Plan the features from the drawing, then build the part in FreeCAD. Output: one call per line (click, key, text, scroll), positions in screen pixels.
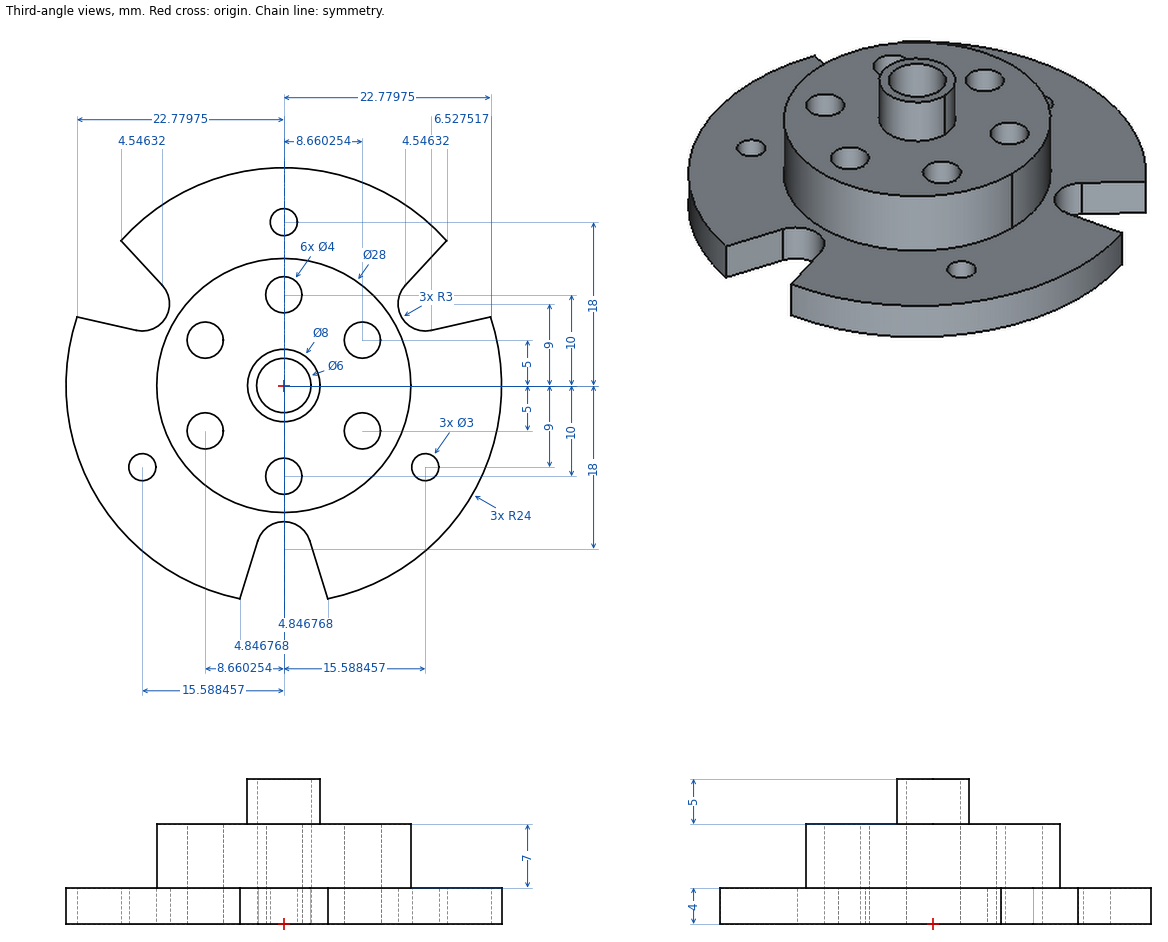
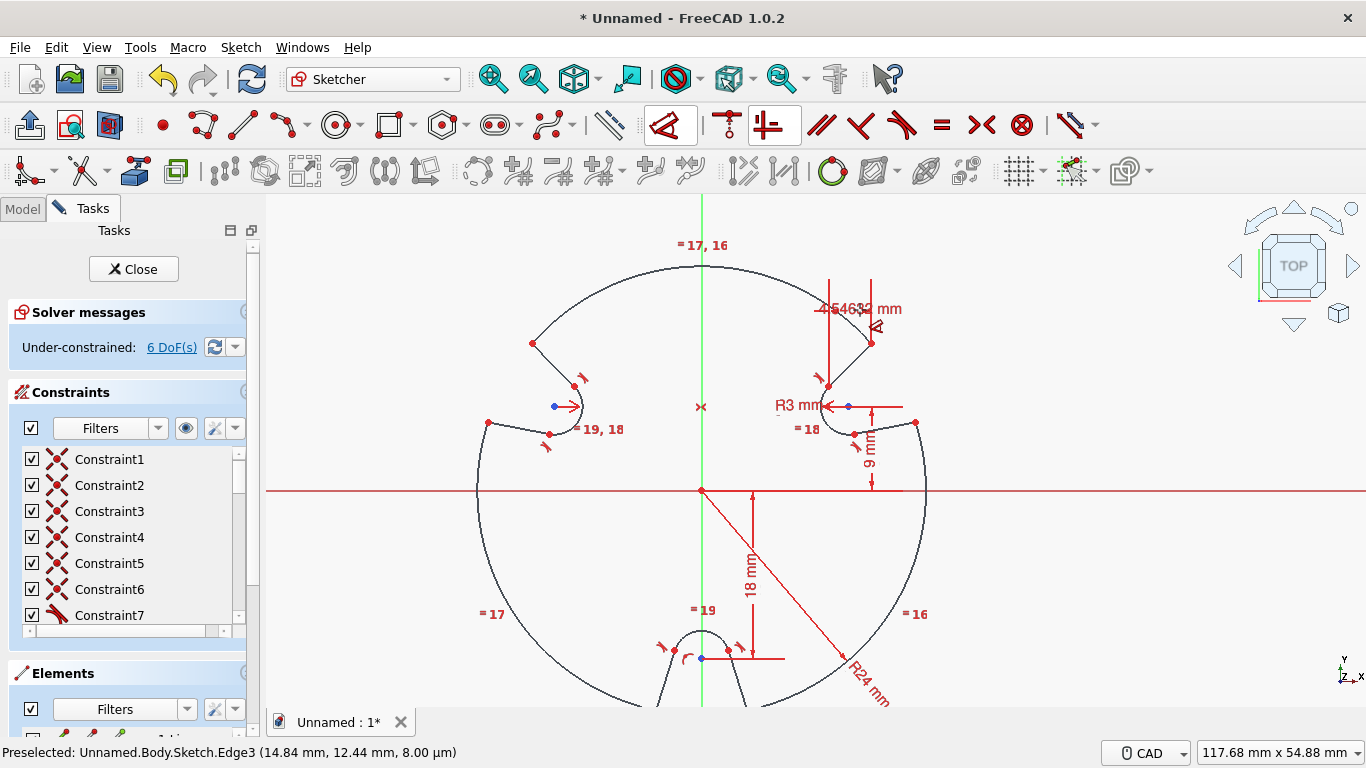
click(545, 357)
click(543, 310)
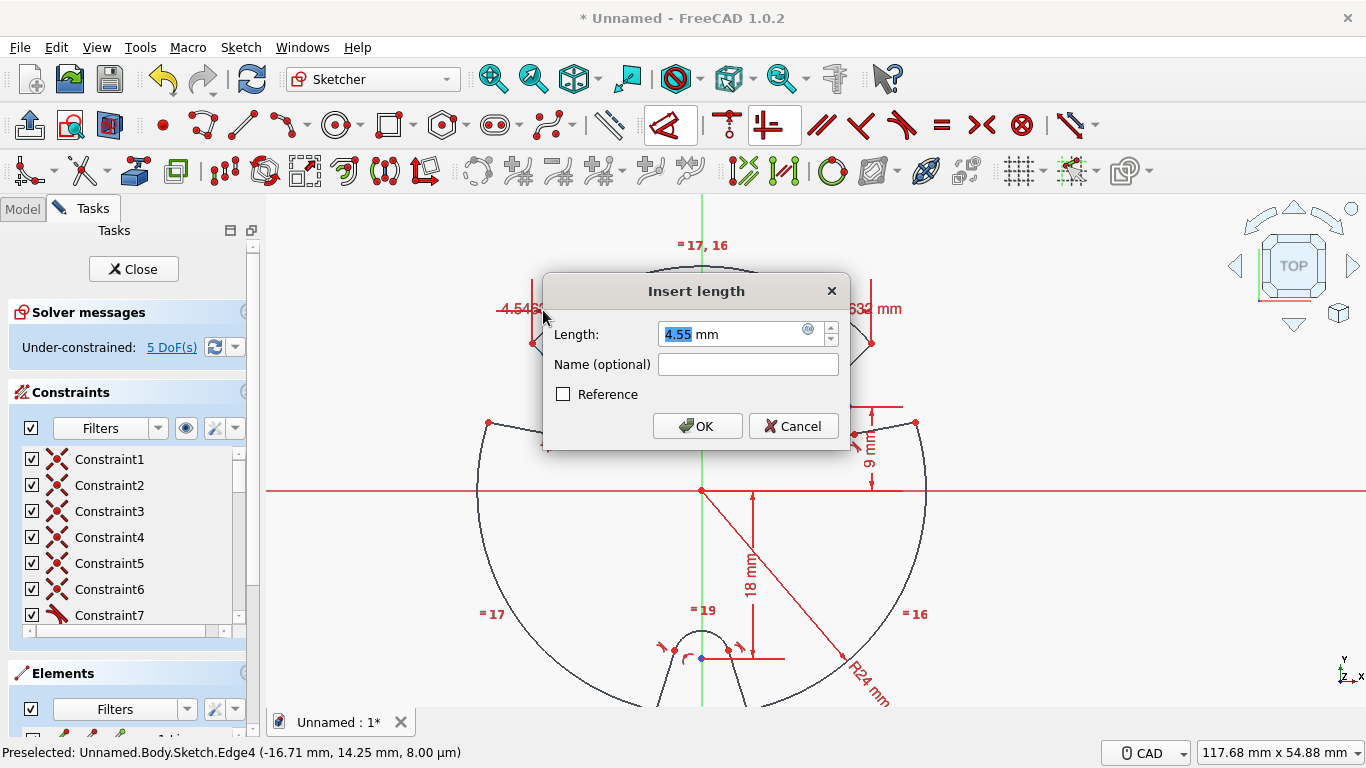
text(4.54632)
key(Return)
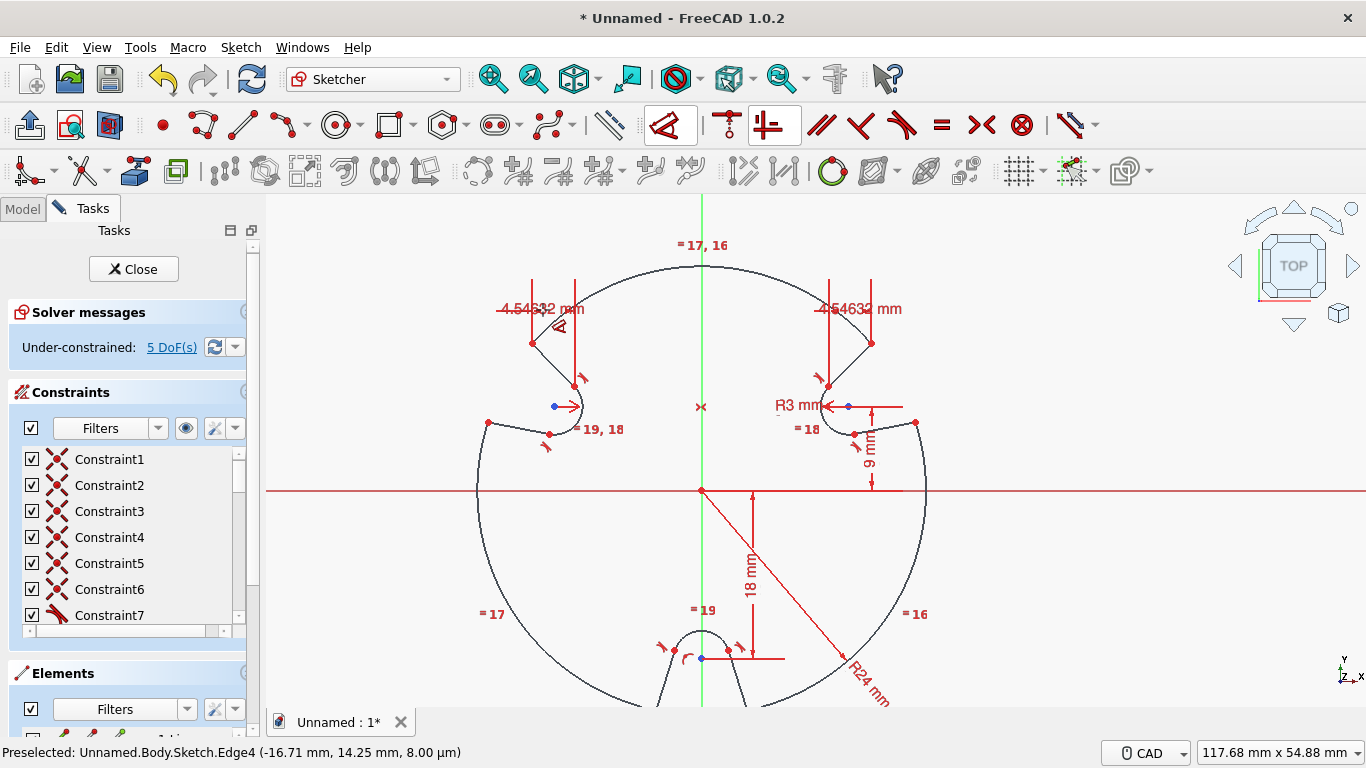
scroll(841, 373, down, 2)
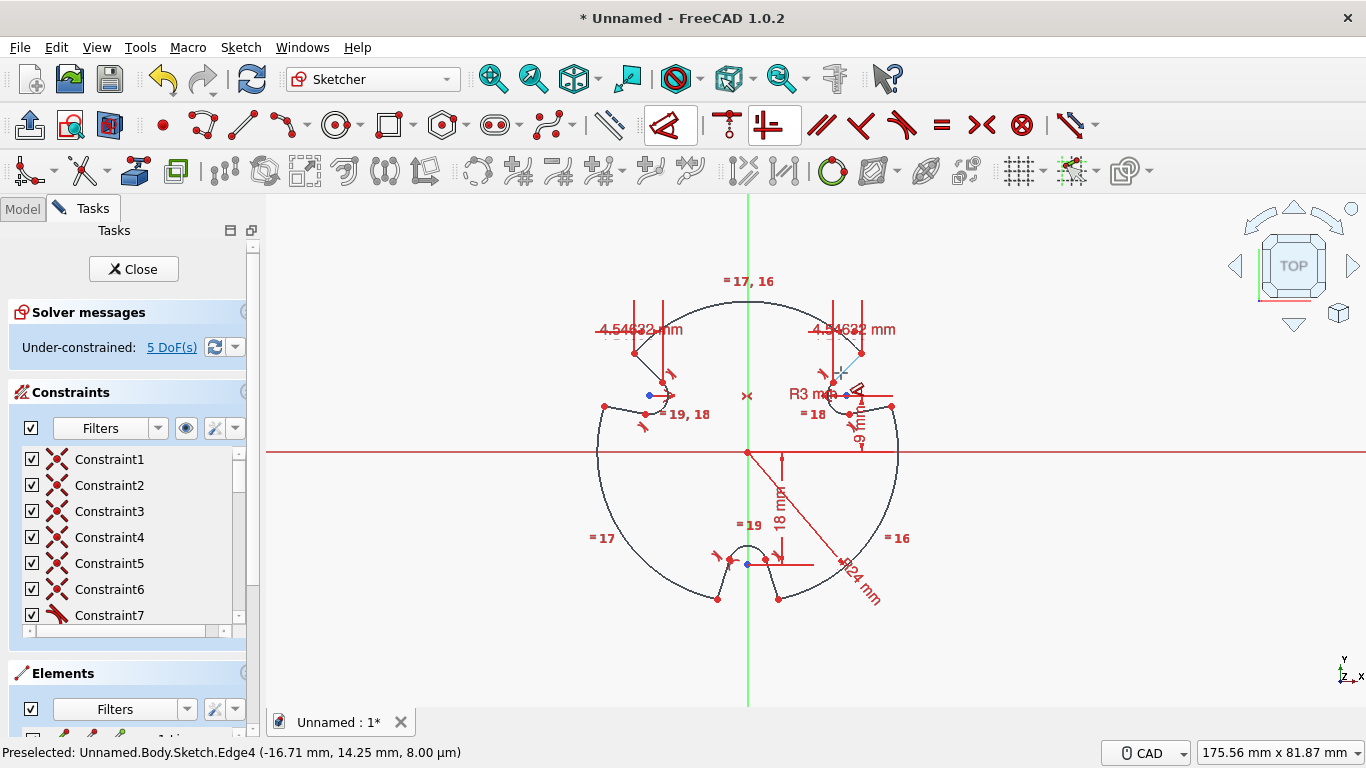
scroll(778, 599, up, 2)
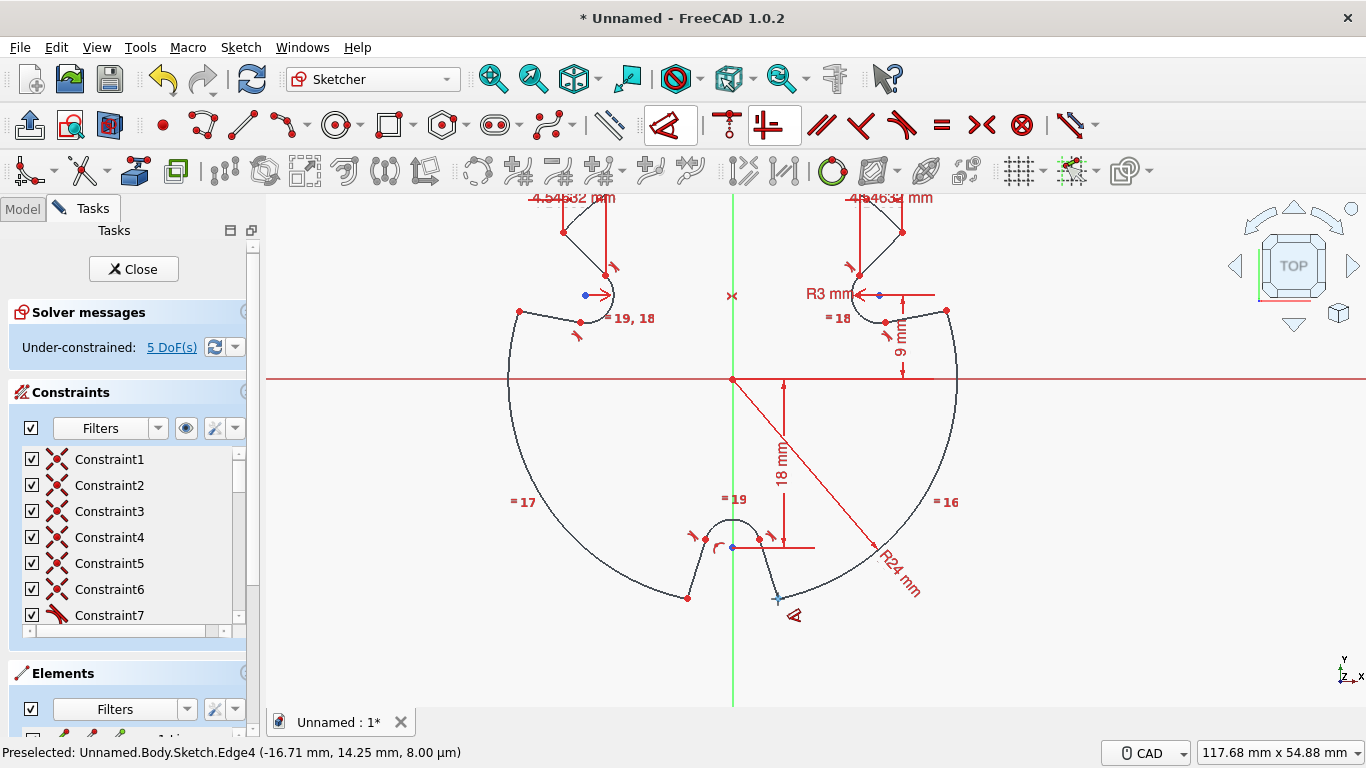
click(778, 599)
click(755, 633)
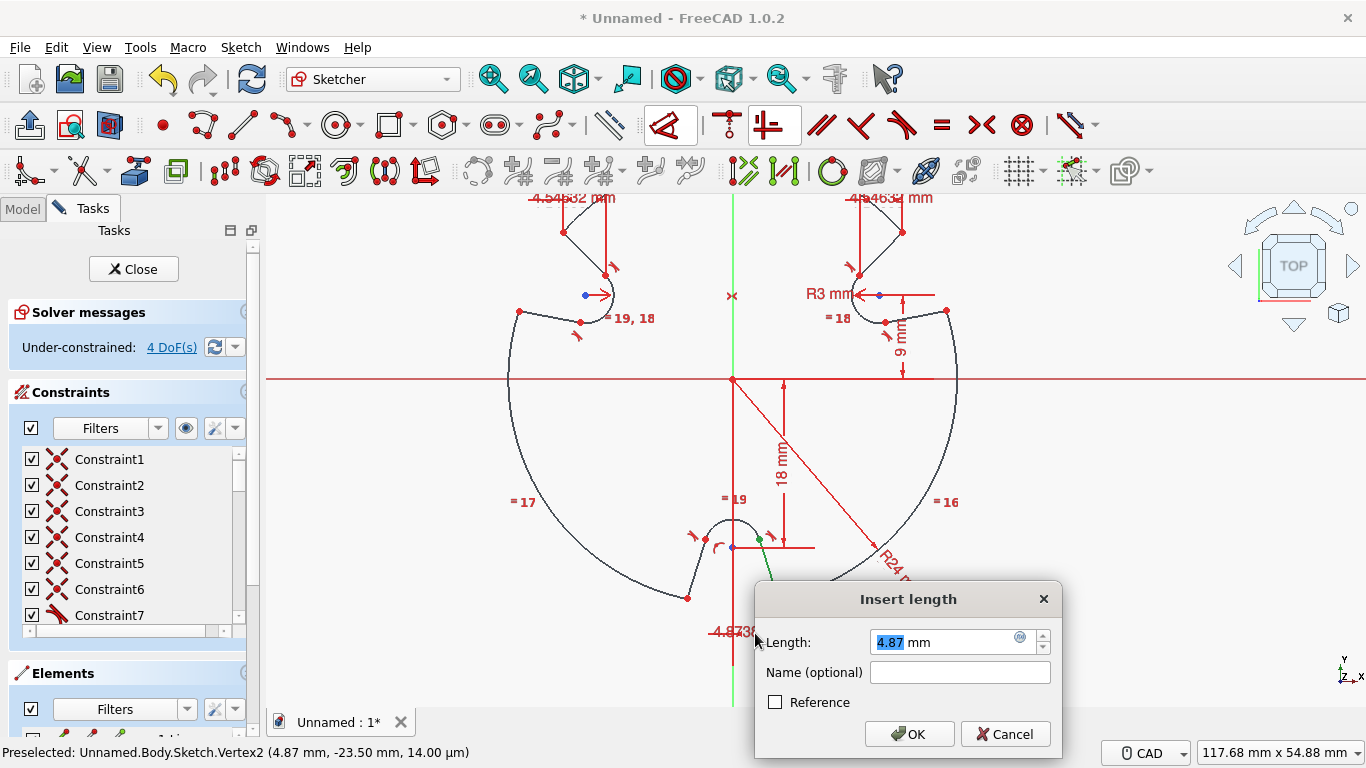
text(4.846768)
key(Return)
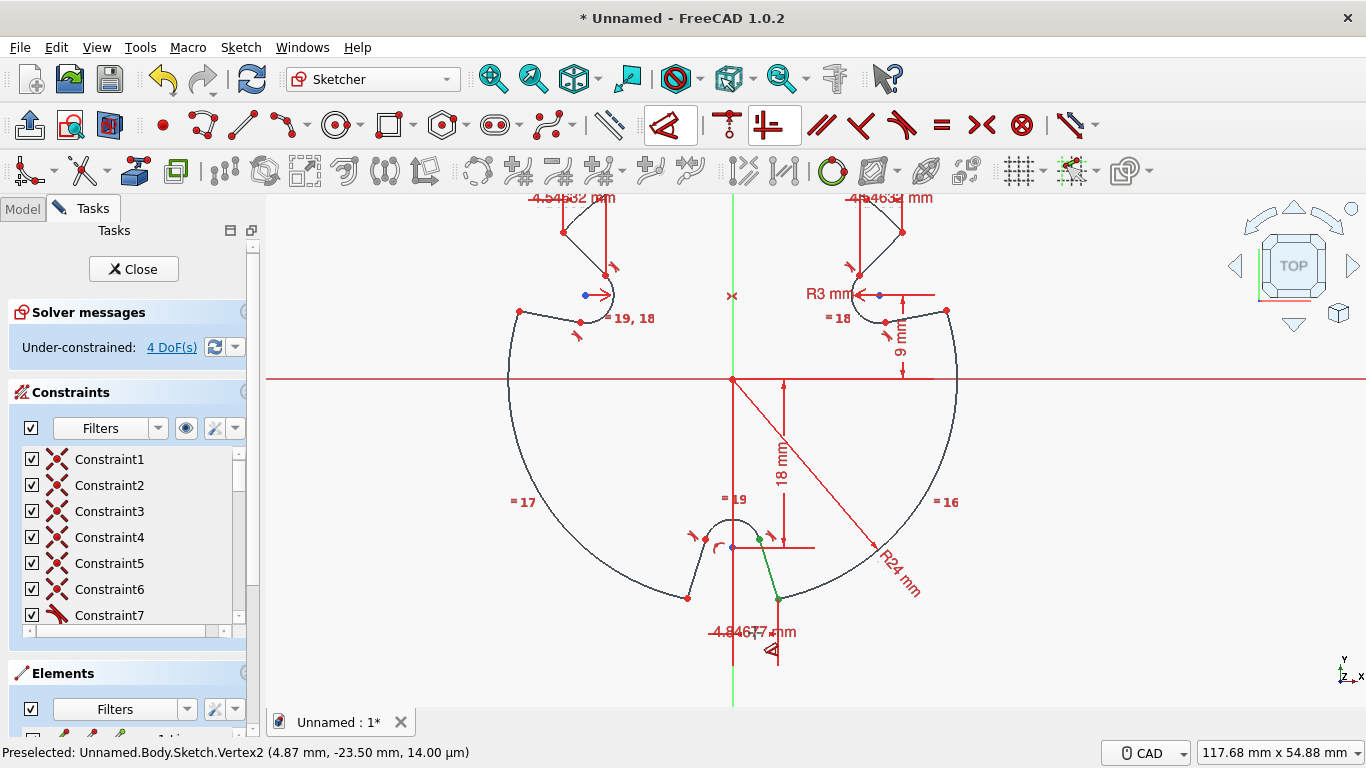
click(946, 311)
click(840, 277)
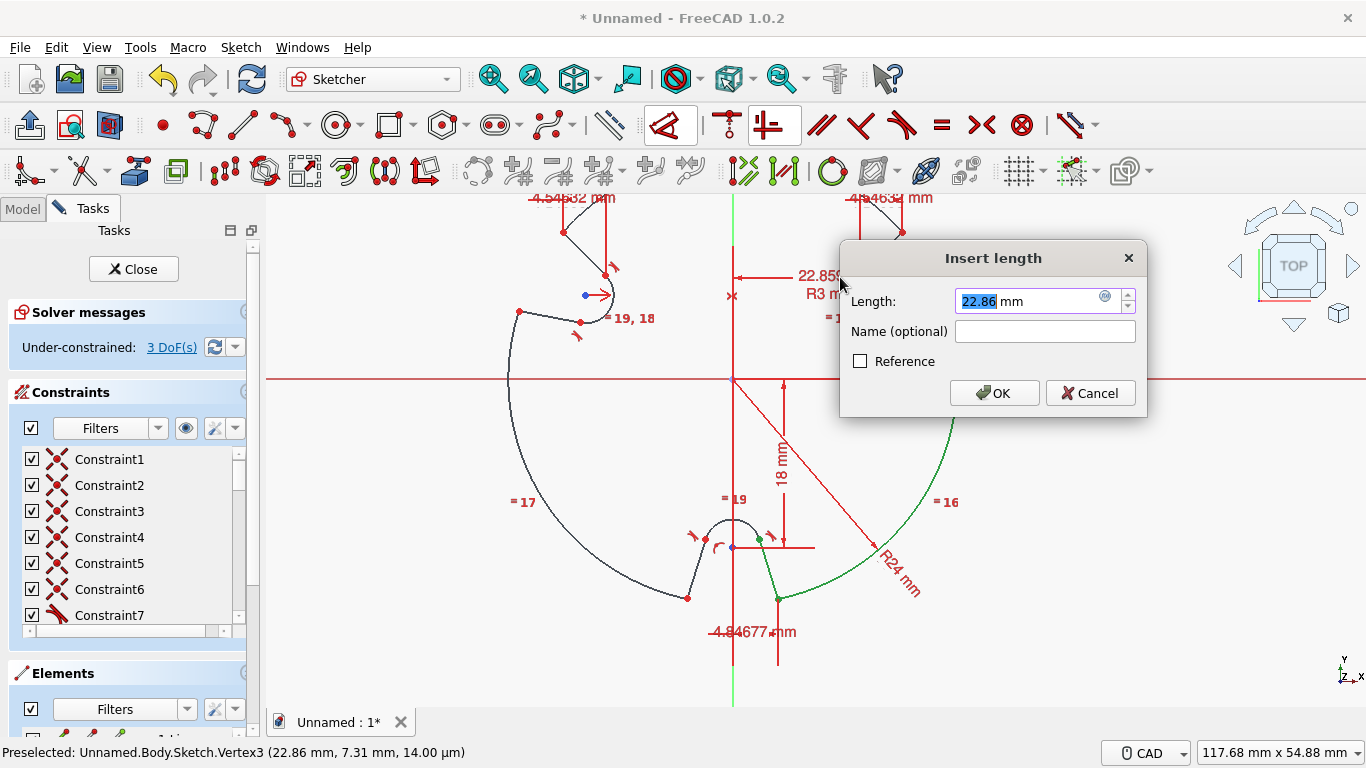
text(22.77975)
key(Return)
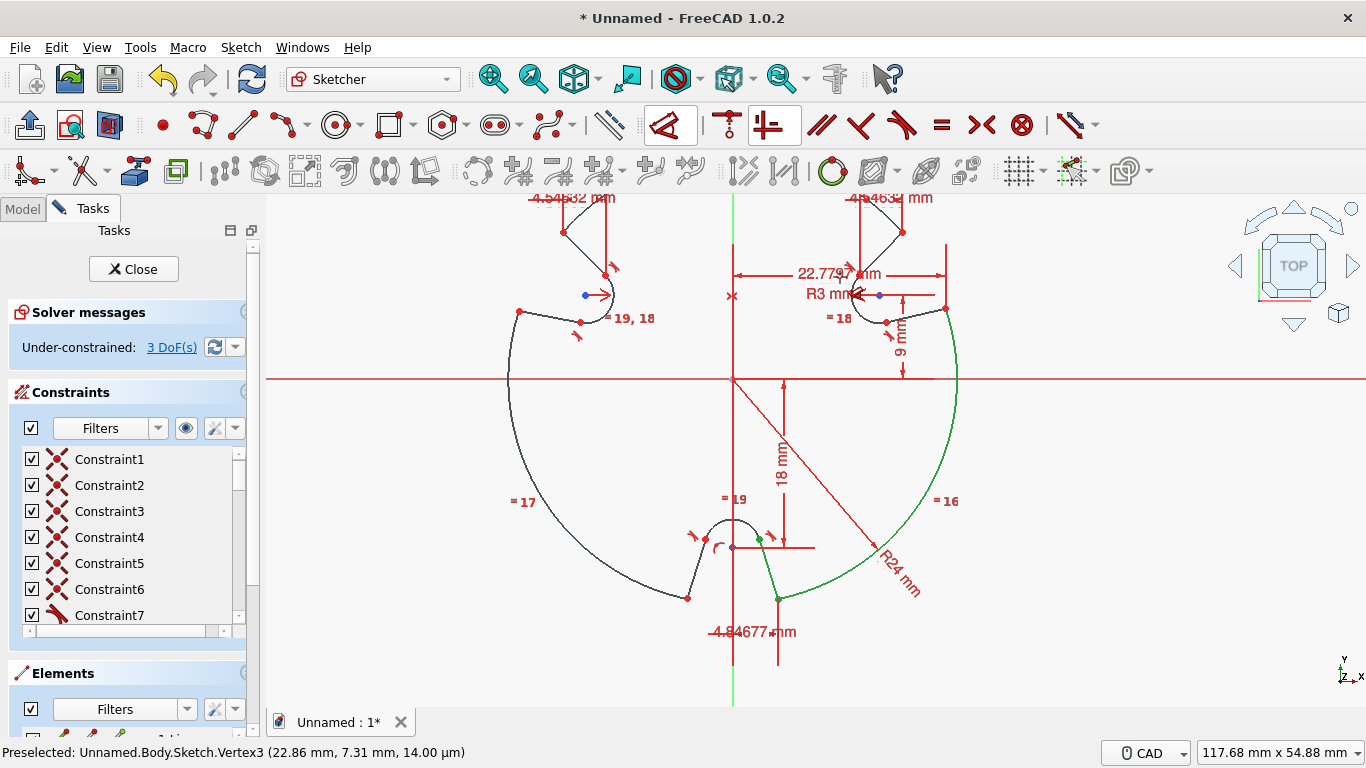
click(519, 311)
click(626, 277)